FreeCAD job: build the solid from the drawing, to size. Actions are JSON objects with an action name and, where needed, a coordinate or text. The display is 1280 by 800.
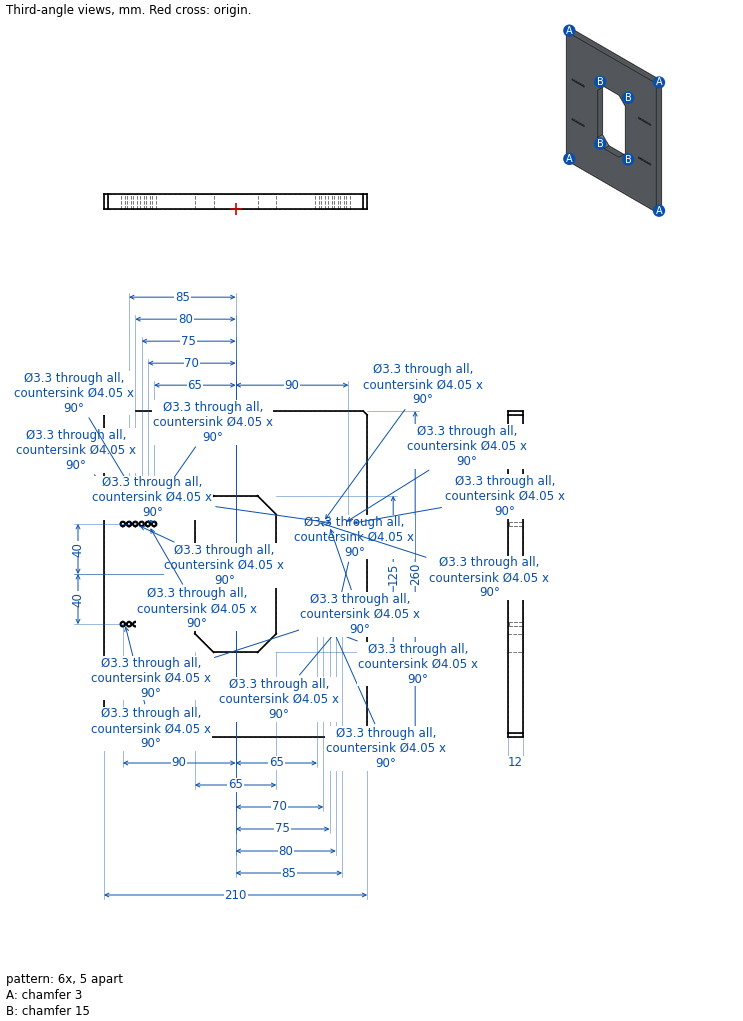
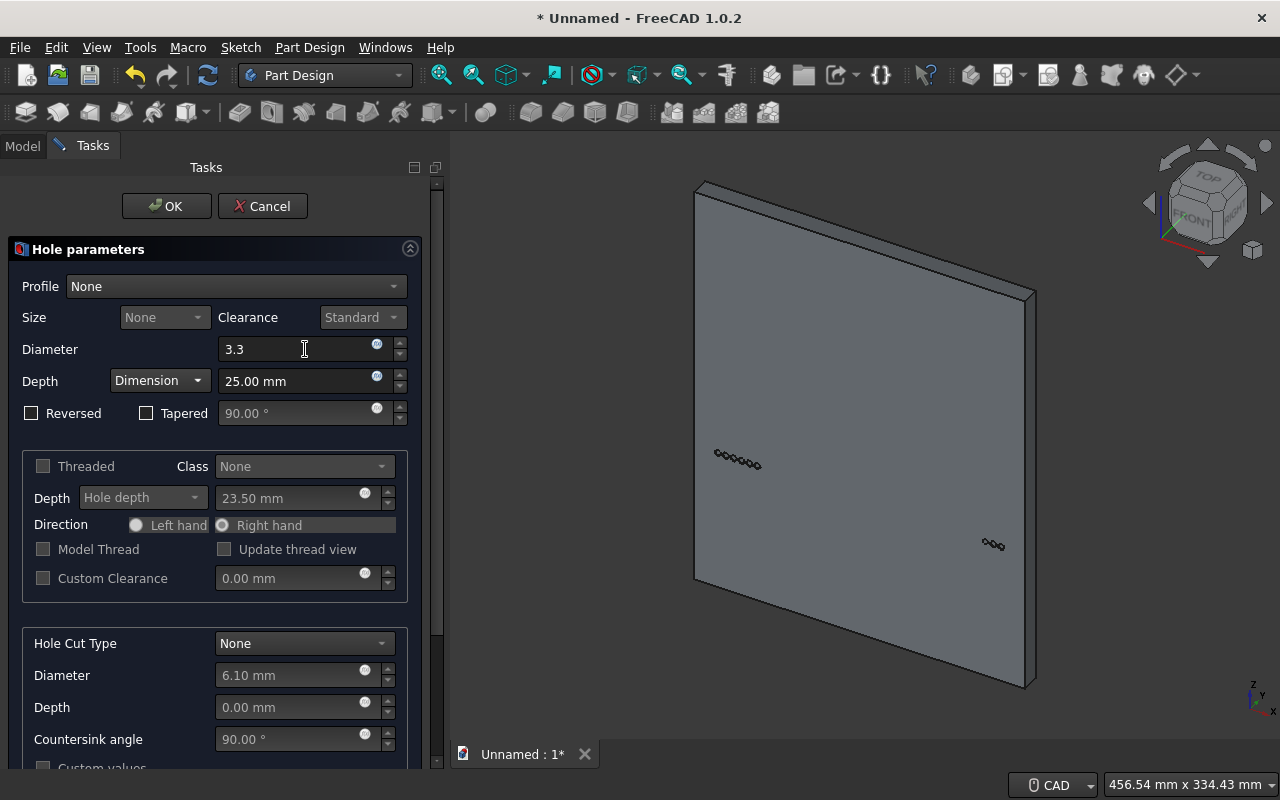
{"action": "left_click", "coordinate": [161, 380]}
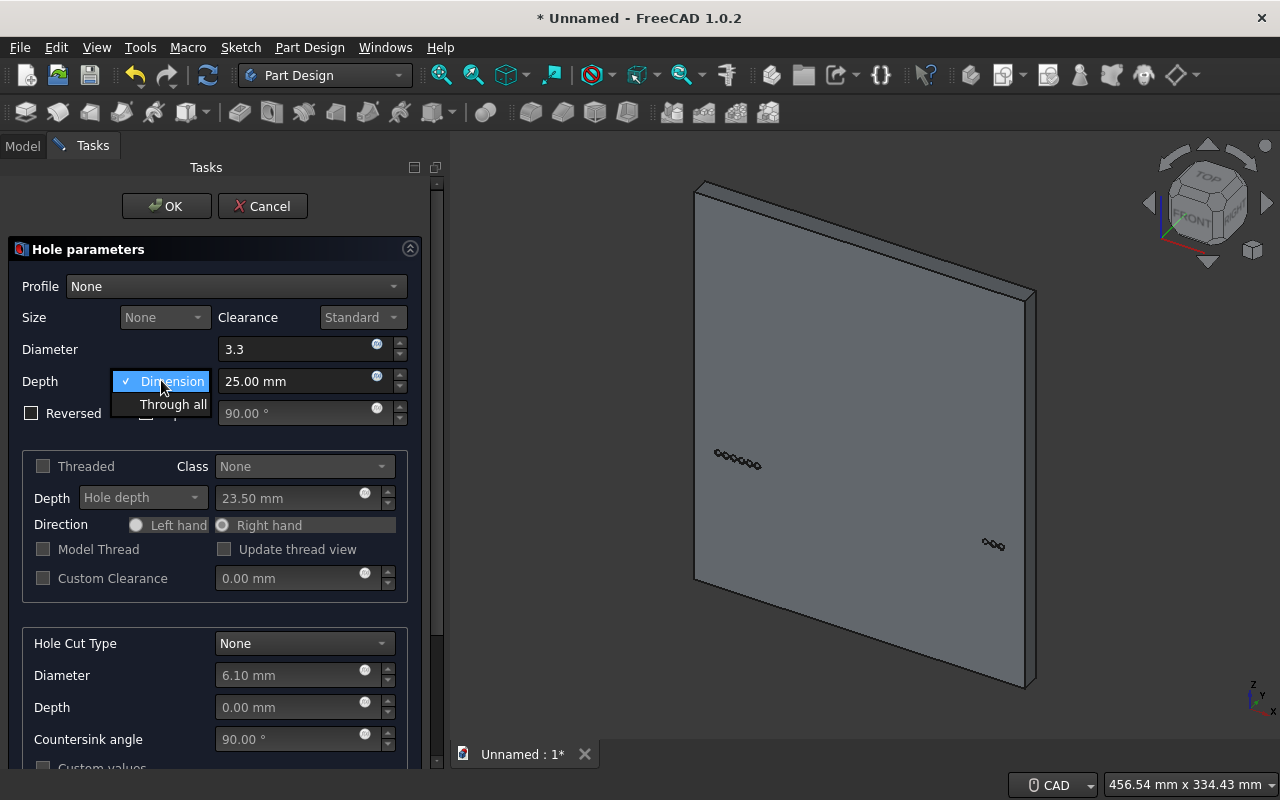
{"action": "left_click", "coordinate": [160, 404]}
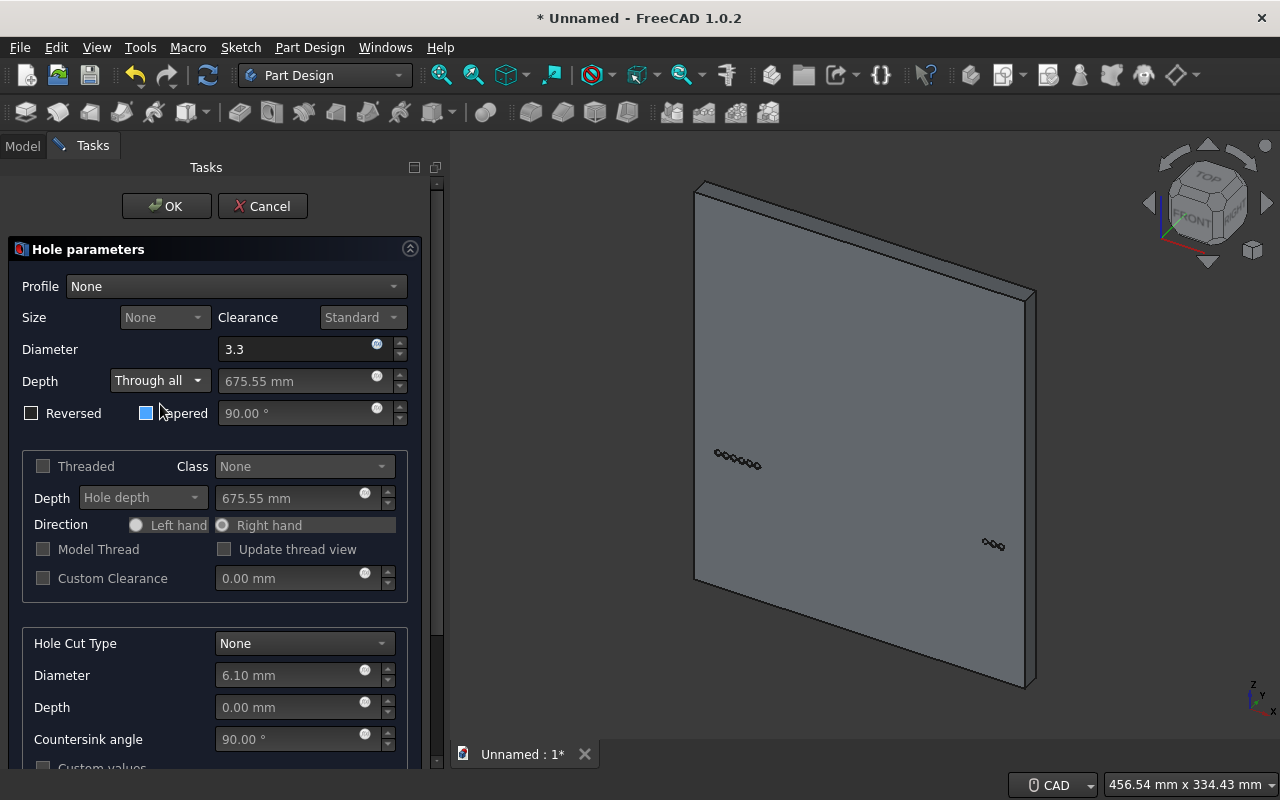
{"action": "left_click", "coordinate": [306, 644]}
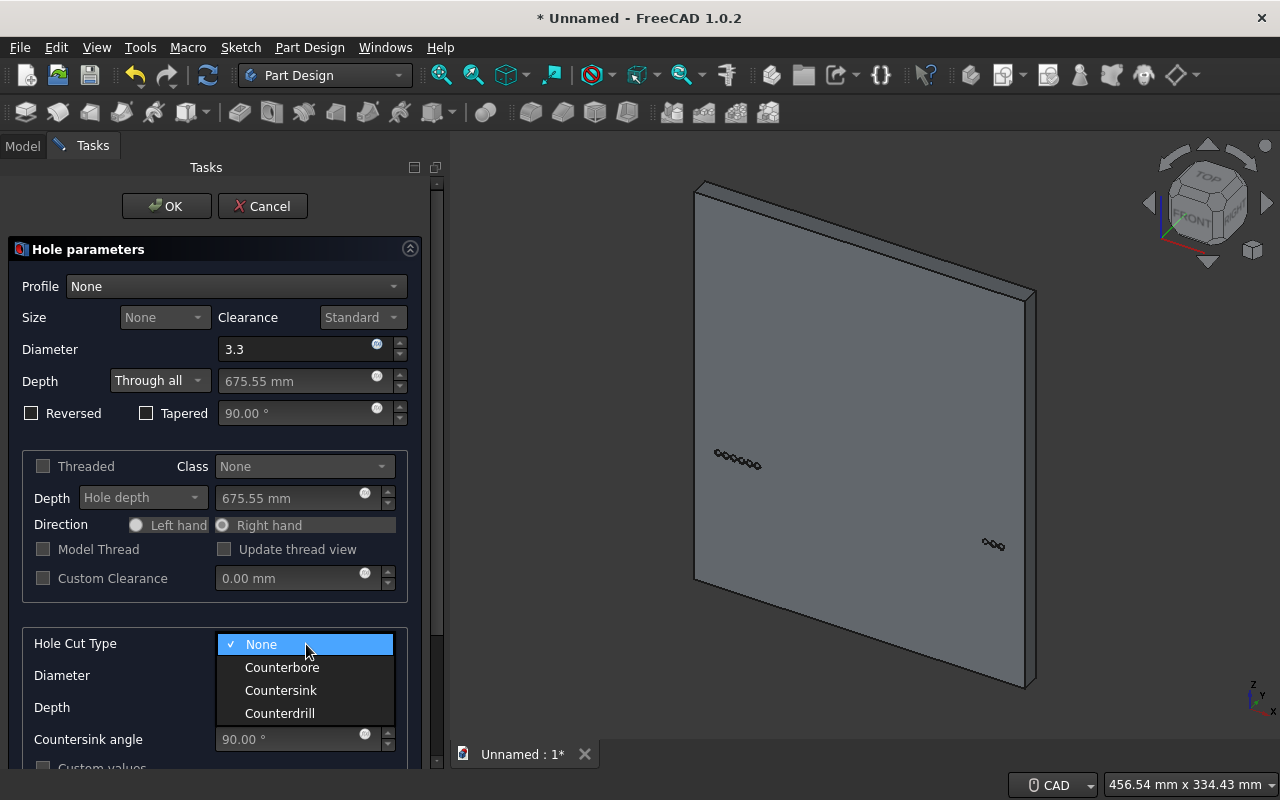
{"action": "left_click", "coordinate": [304, 690]}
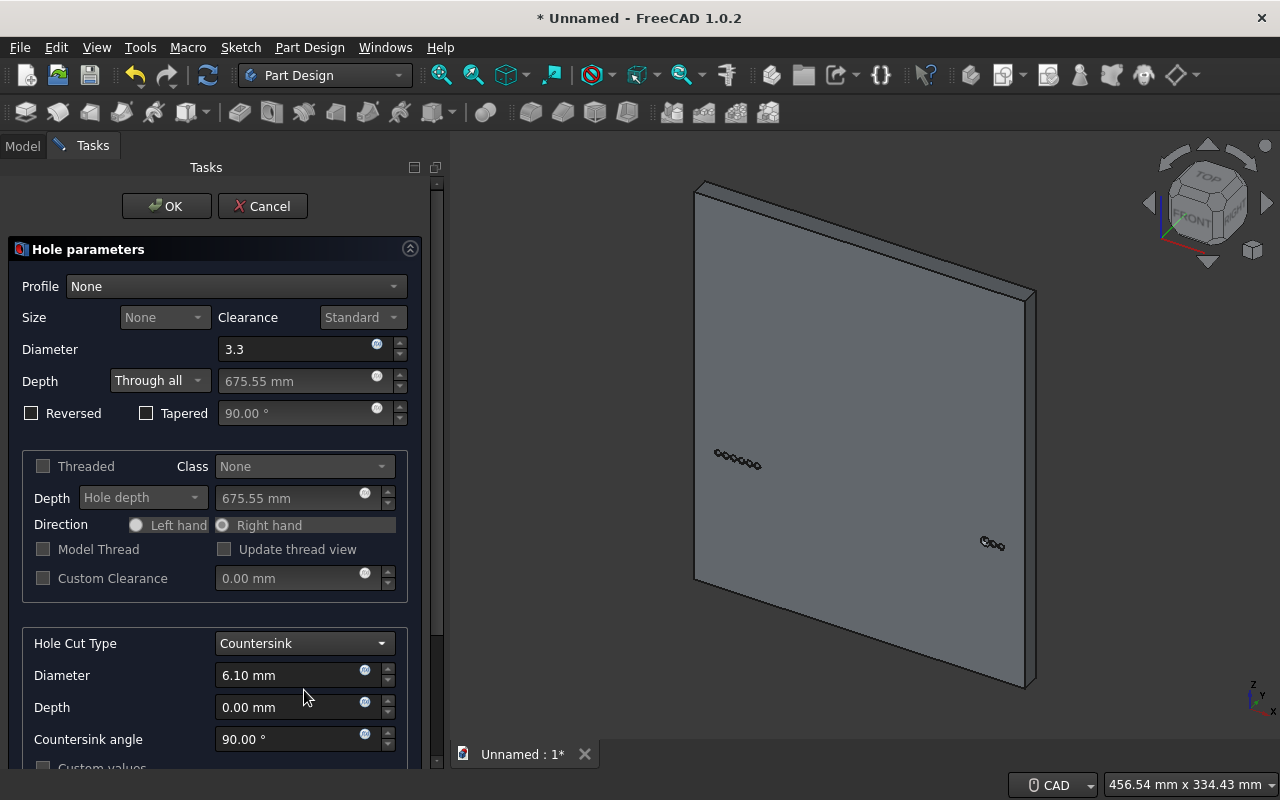
{"action": "triple_click", "coordinate": [298, 675]}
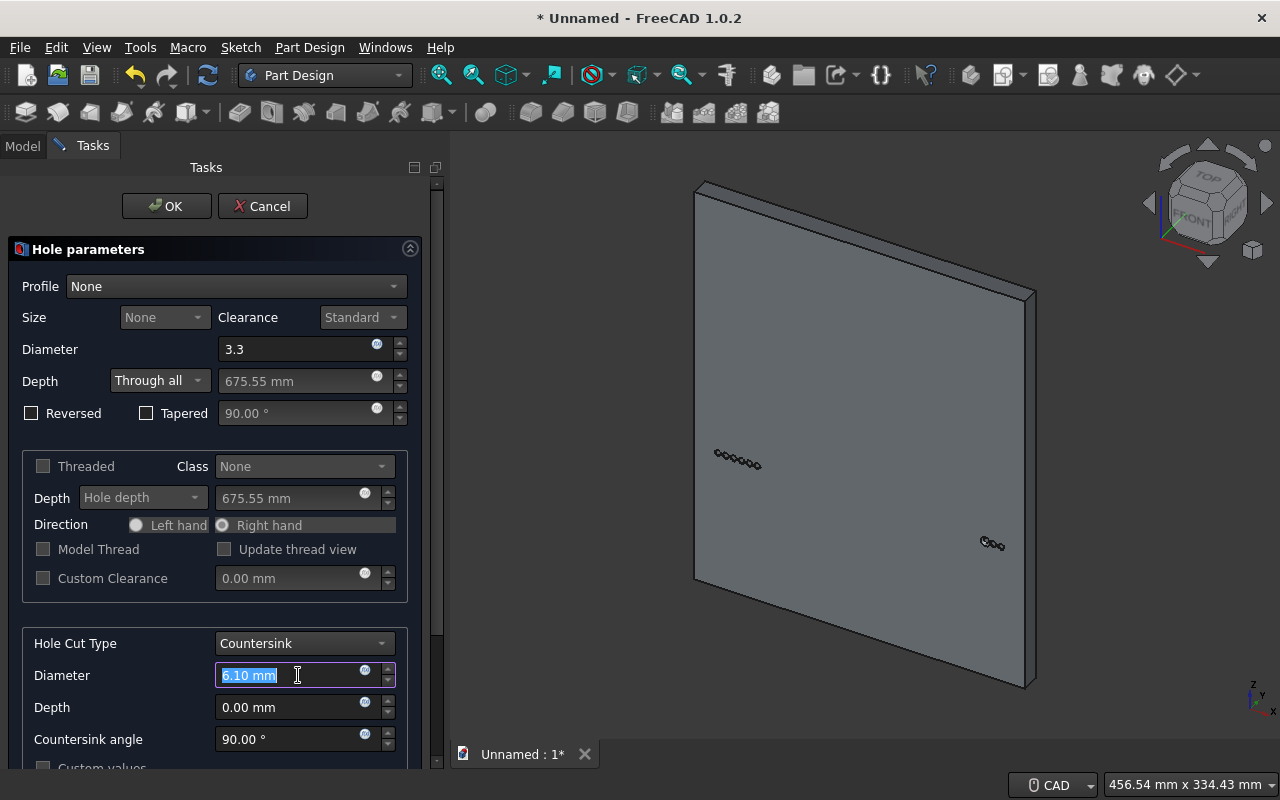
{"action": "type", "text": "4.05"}
{"action": "key", "text": "Tab"}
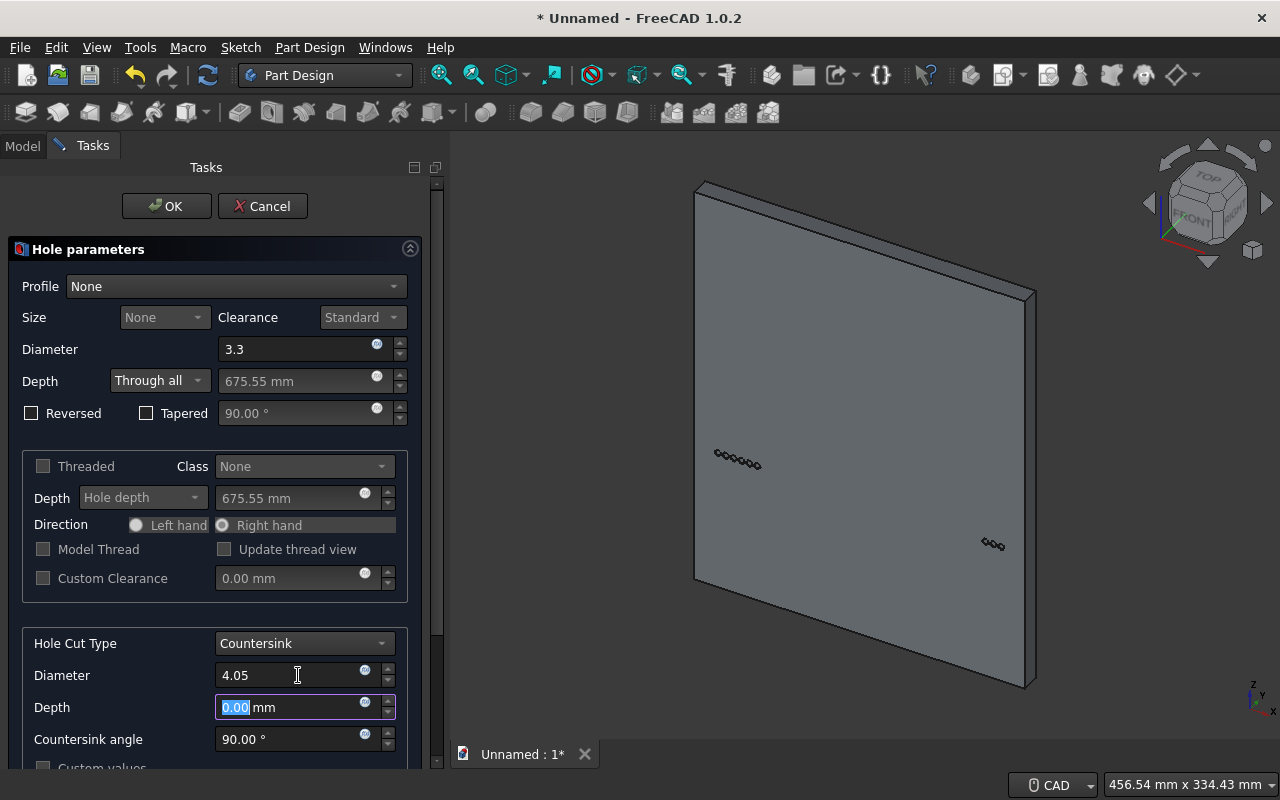
{"action": "left_click", "coordinate": [167, 206]}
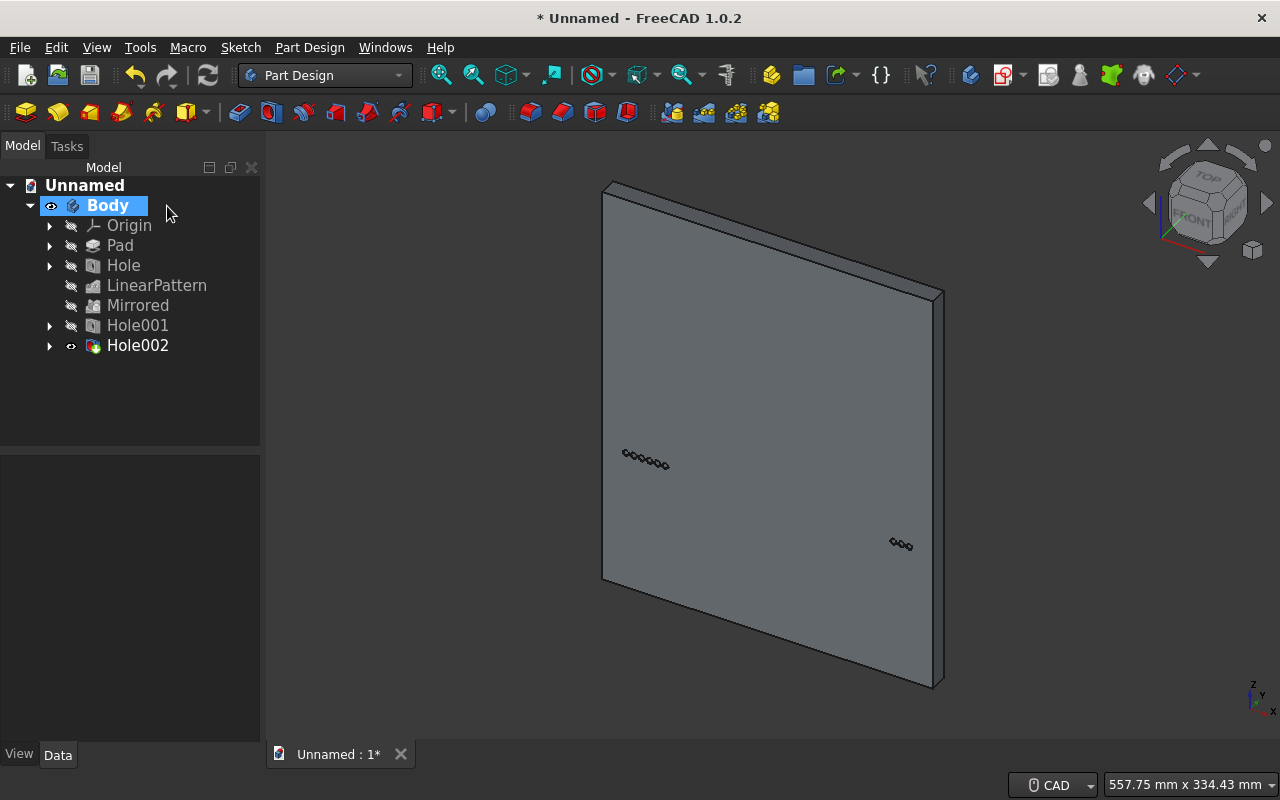
{"action": "left_click", "coordinate": [768, 384]}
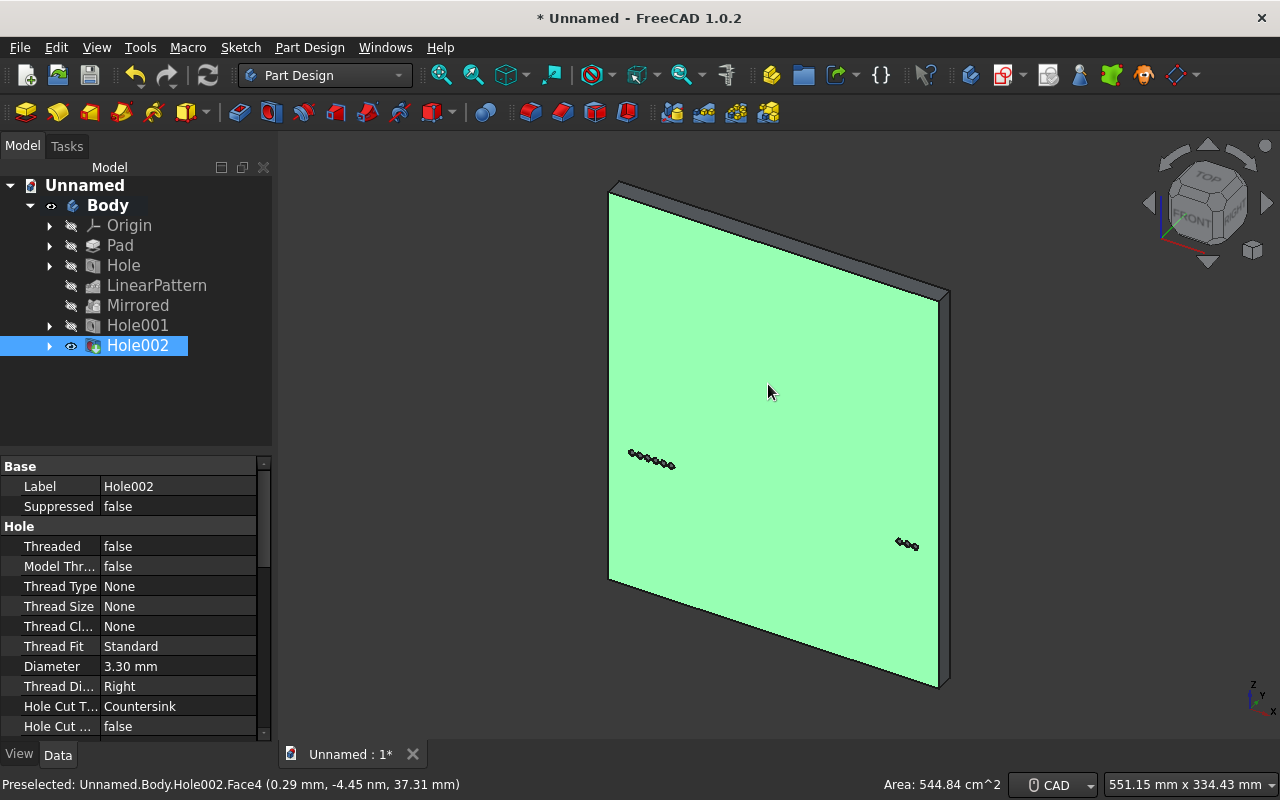
{"action": "left_click", "coordinate": [1004, 76]}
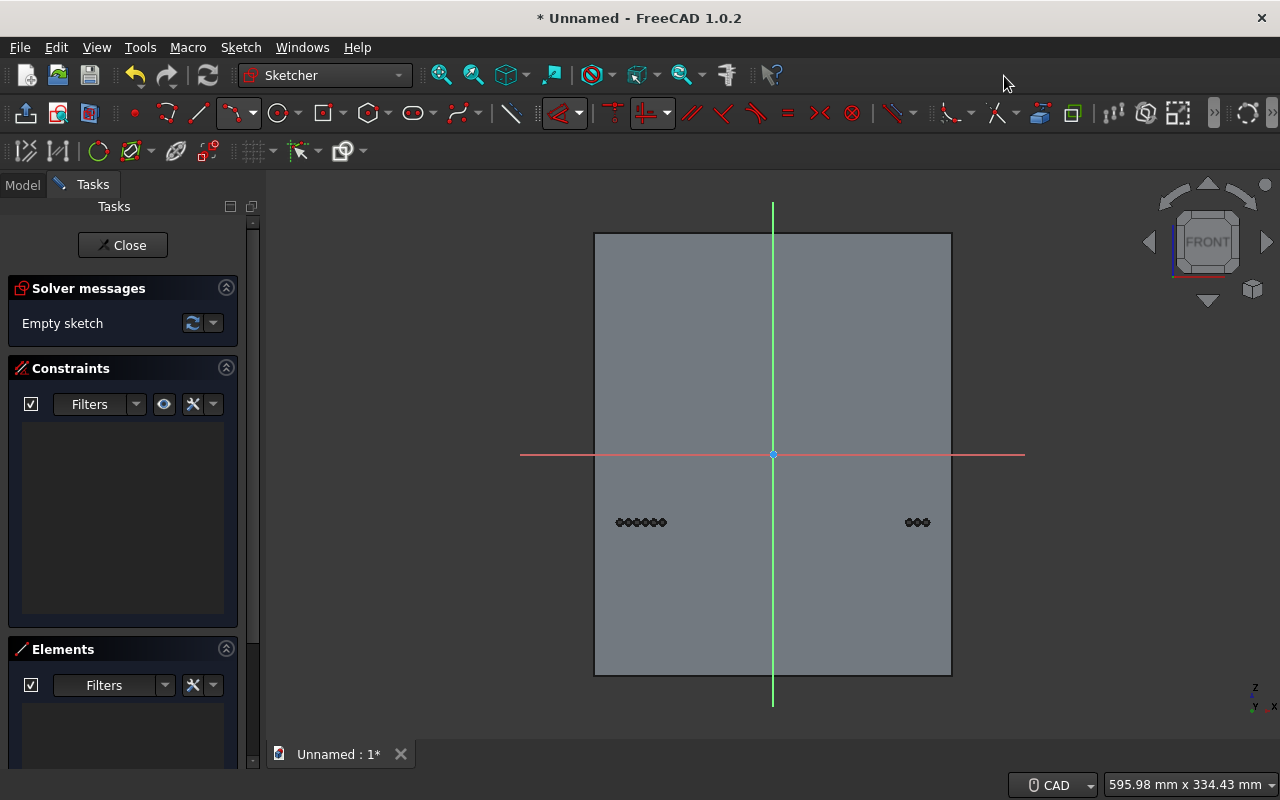
{"action": "scroll", "coordinate": [911, 526], "scroll_direction": "up", "scroll_amount": 15}